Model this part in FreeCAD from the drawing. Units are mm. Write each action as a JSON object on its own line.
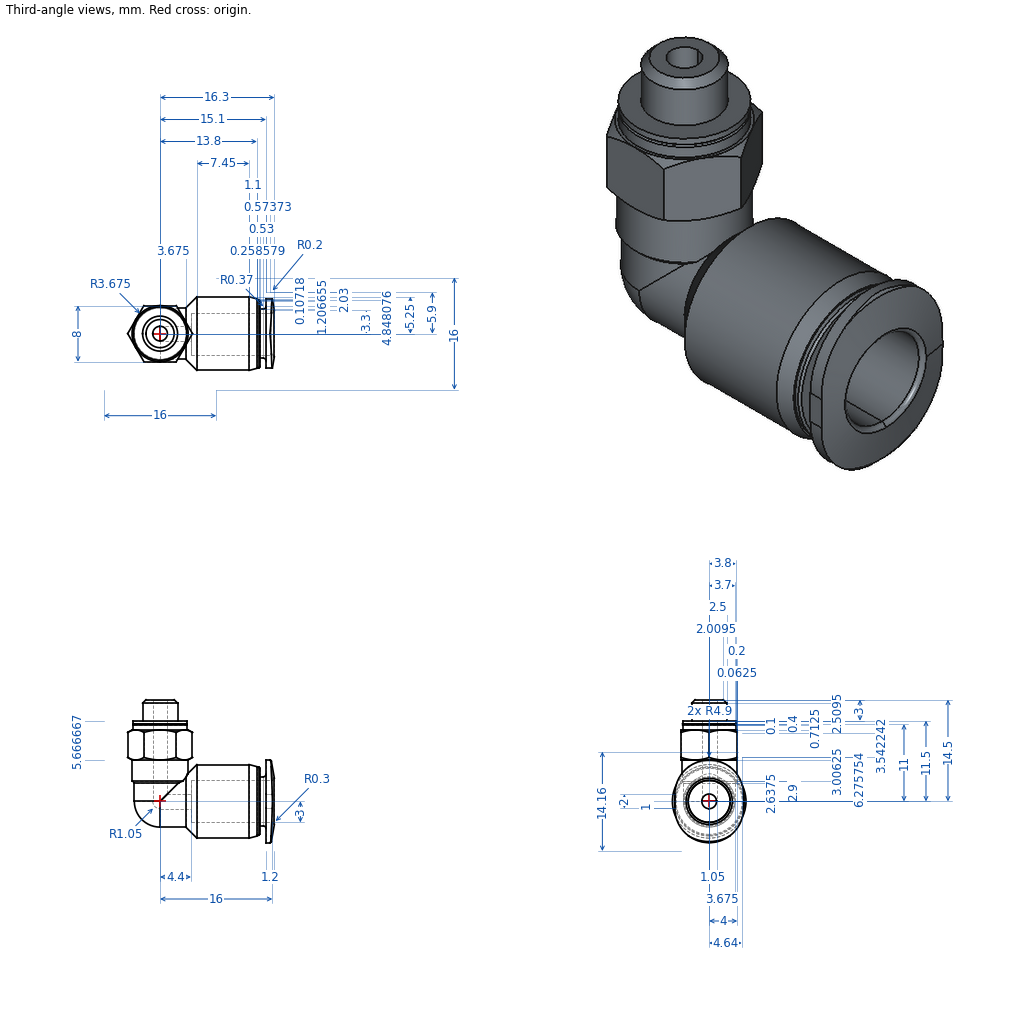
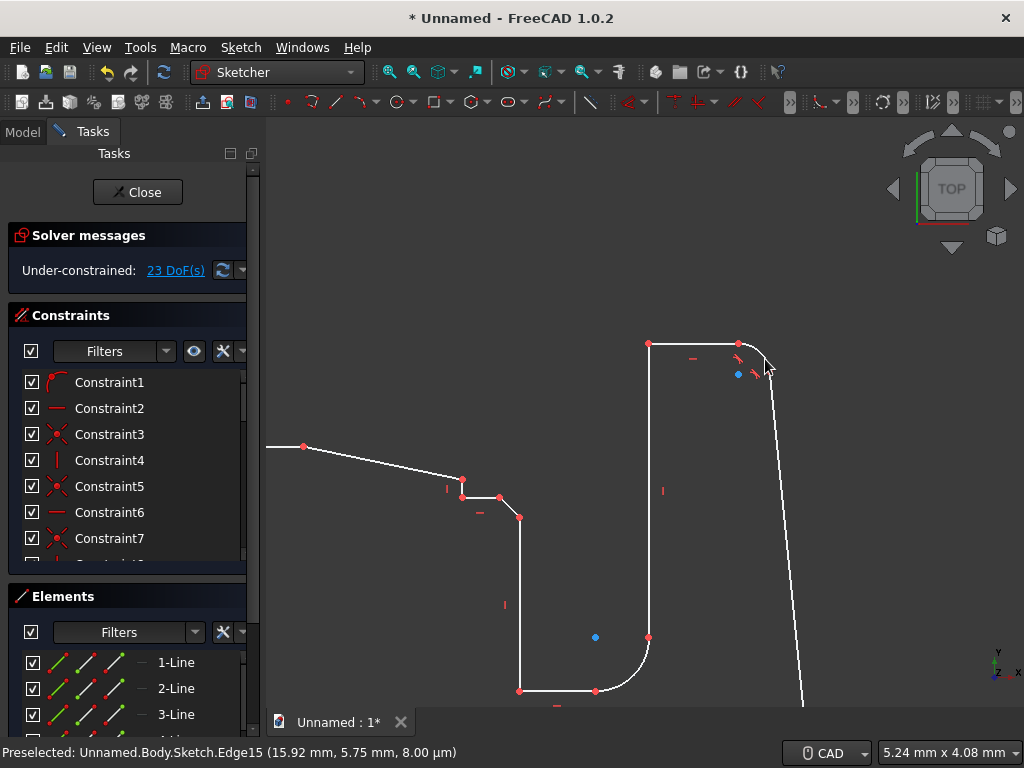
{"action": "scroll", "coordinate": [764, 356], "scroll_direction": "down", "scroll_amount": 10}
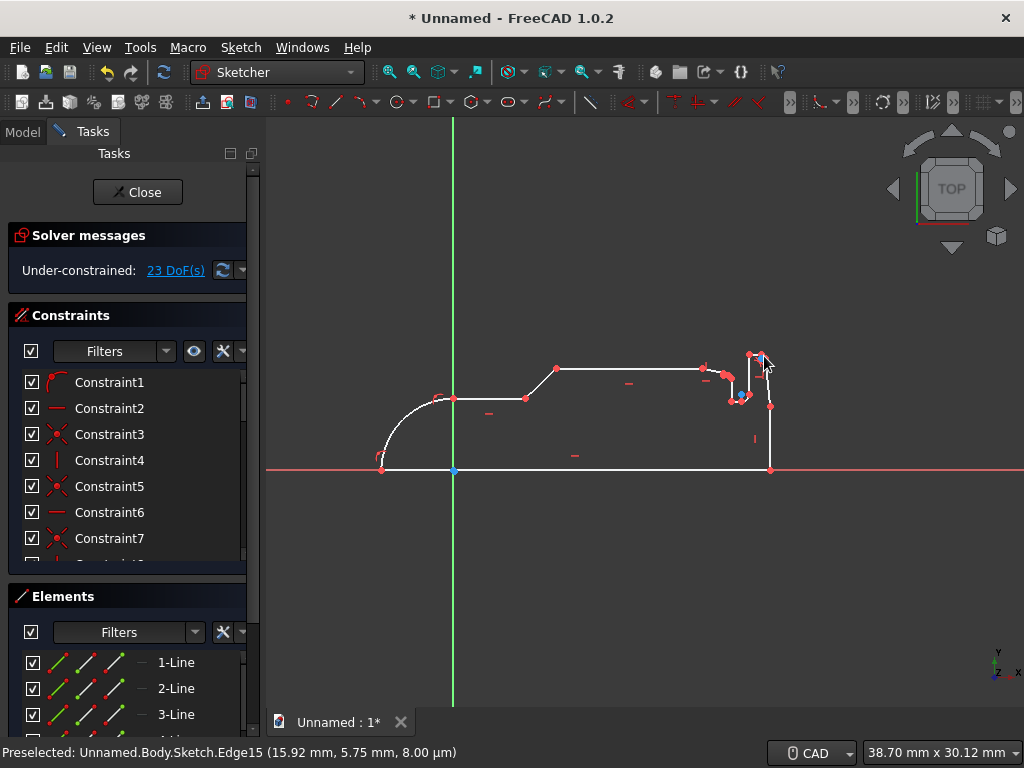
{"action": "left_click", "coordinate": [749, 367]}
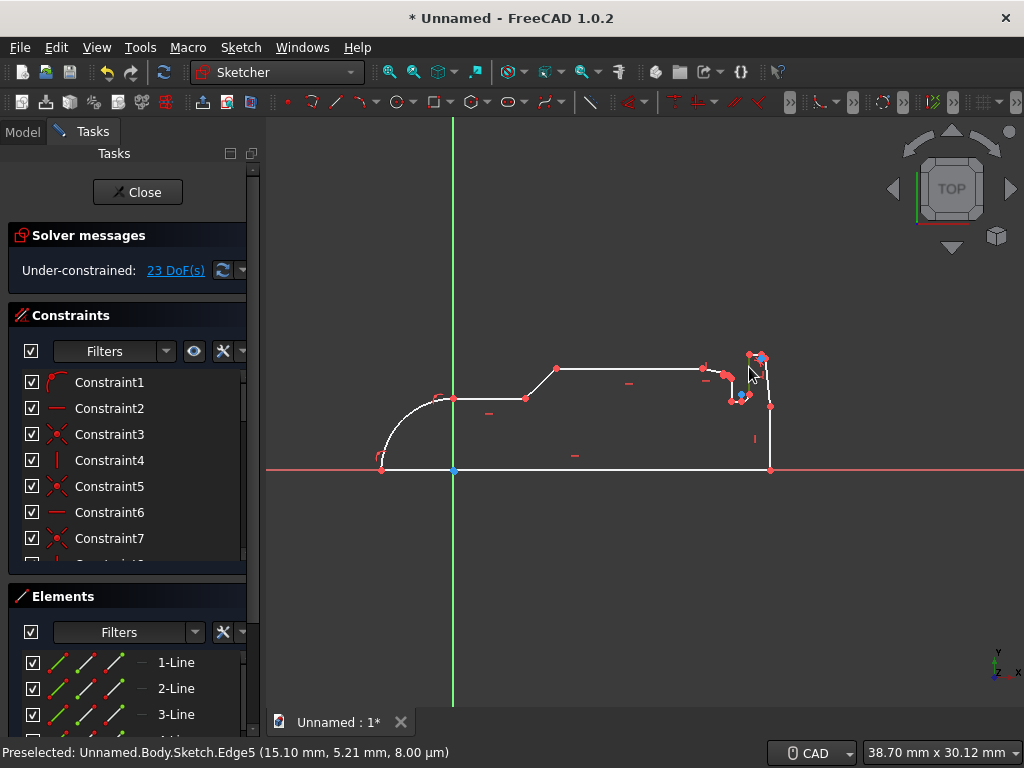
{"action": "scroll", "coordinate": [747, 400], "scroll_direction": "up", "scroll_amount": 5}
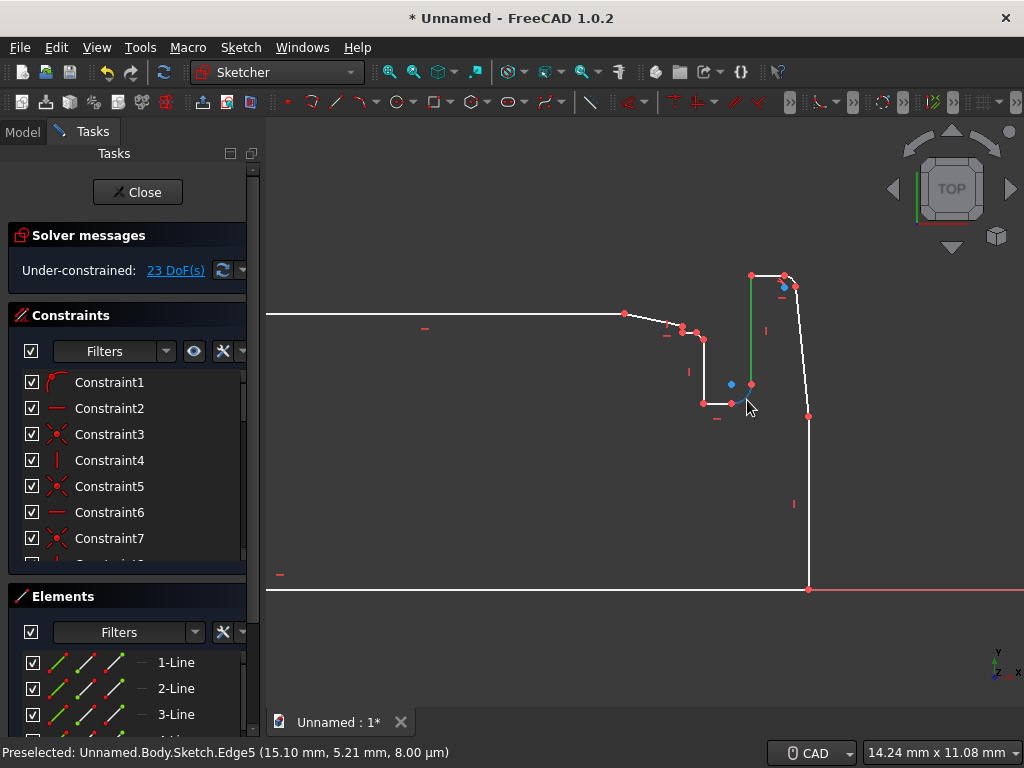
{"action": "left_click", "coordinate": [746, 398]}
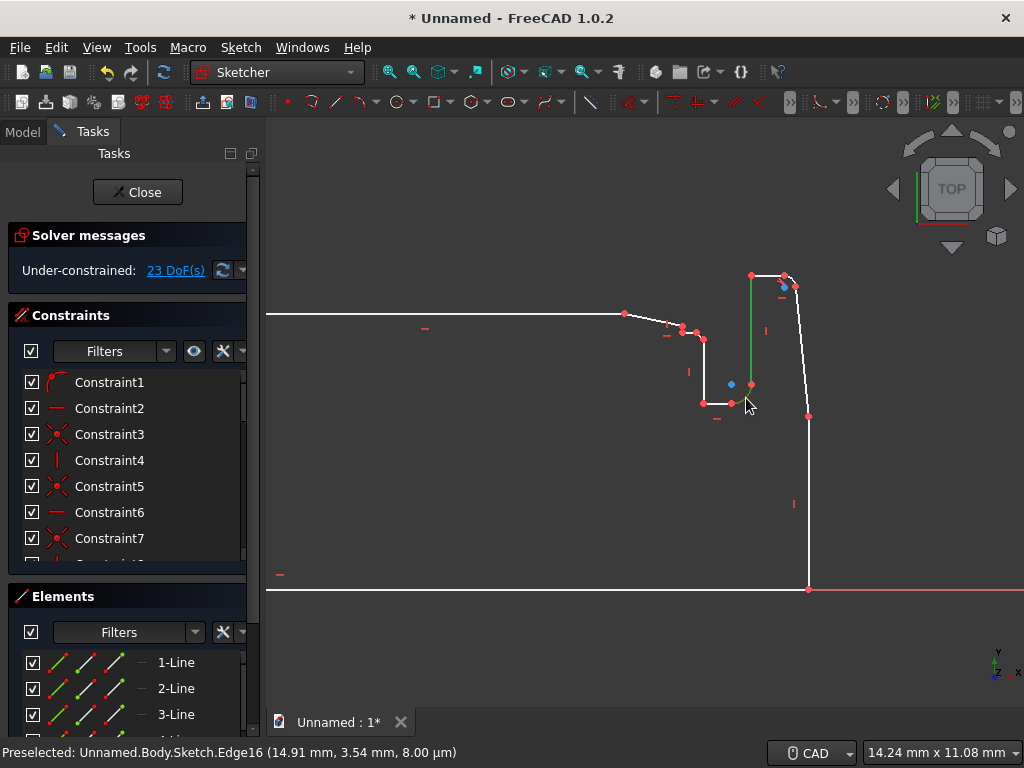
{"action": "key", "text": "t"}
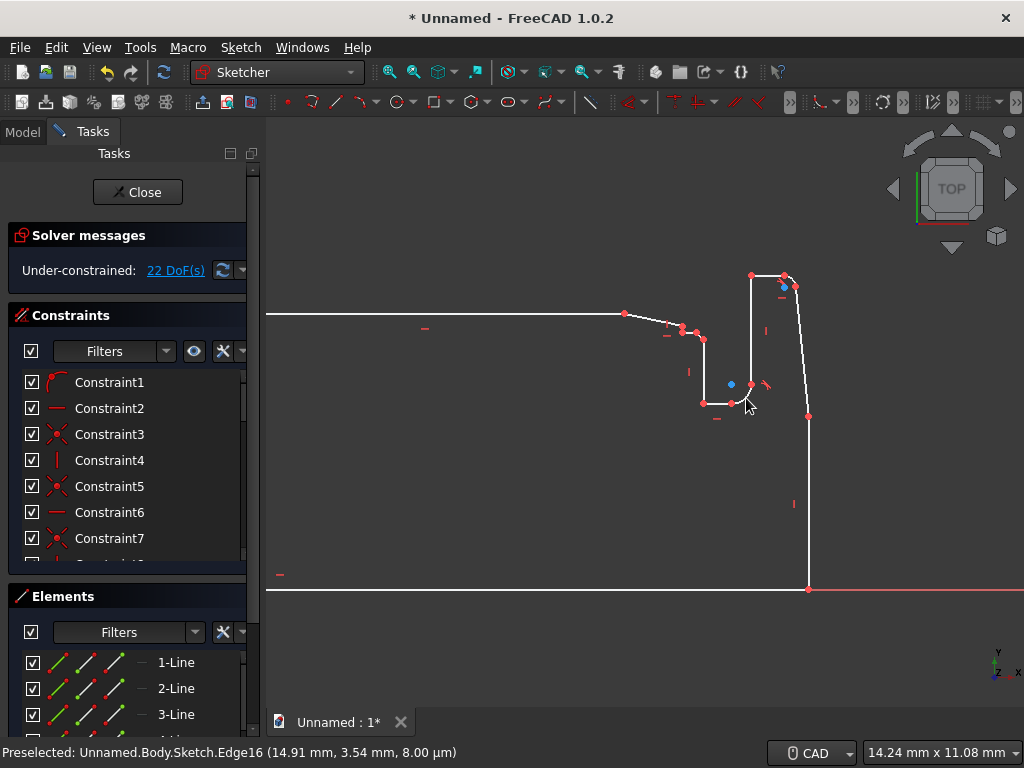
{"action": "scroll", "coordinate": [721, 404], "scroll_direction": "up", "scroll_amount": 2}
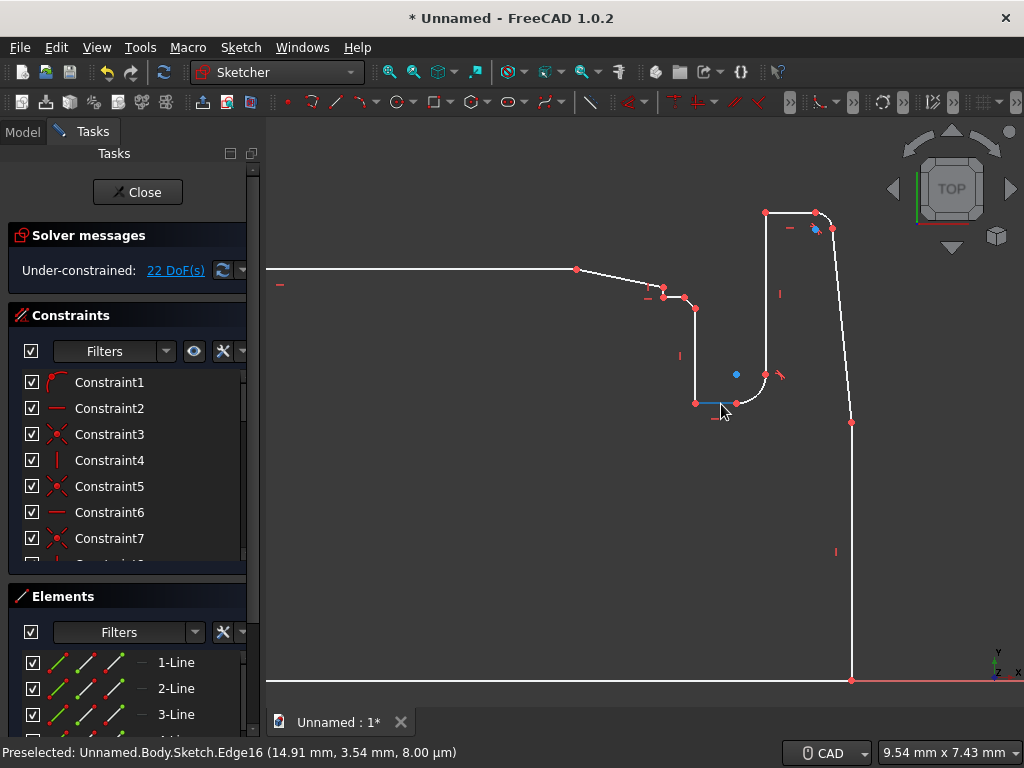
{"action": "left_click", "coordinate": [720, 403]}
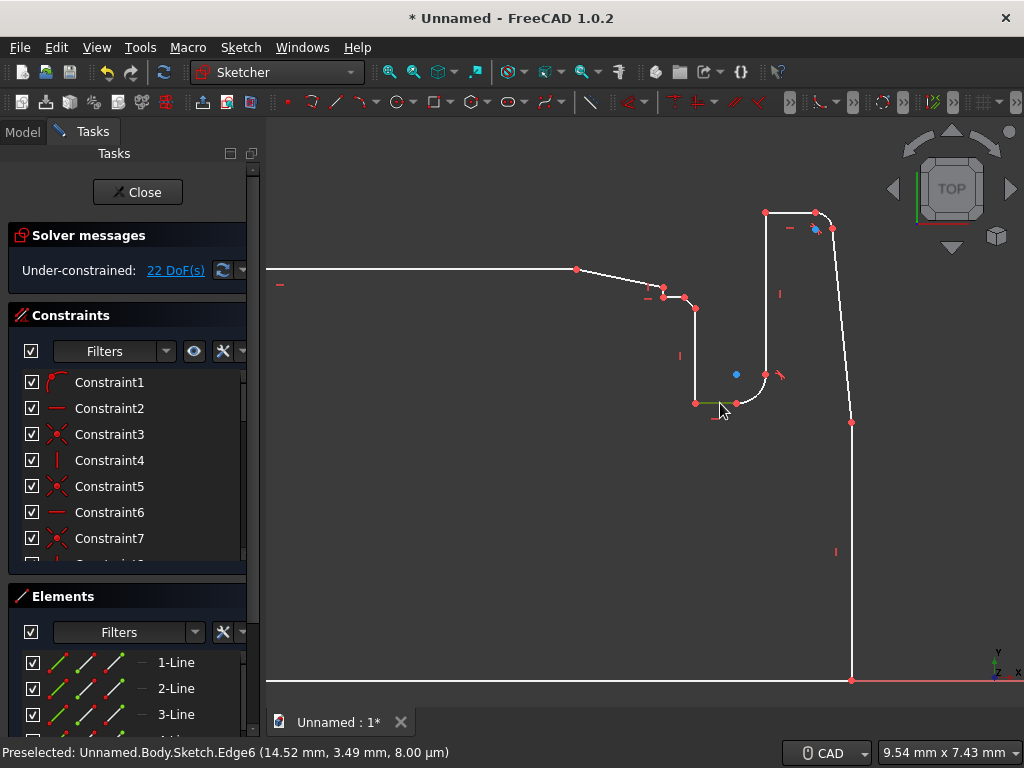
{"action": "left_click", "coordinate": [750, 400]}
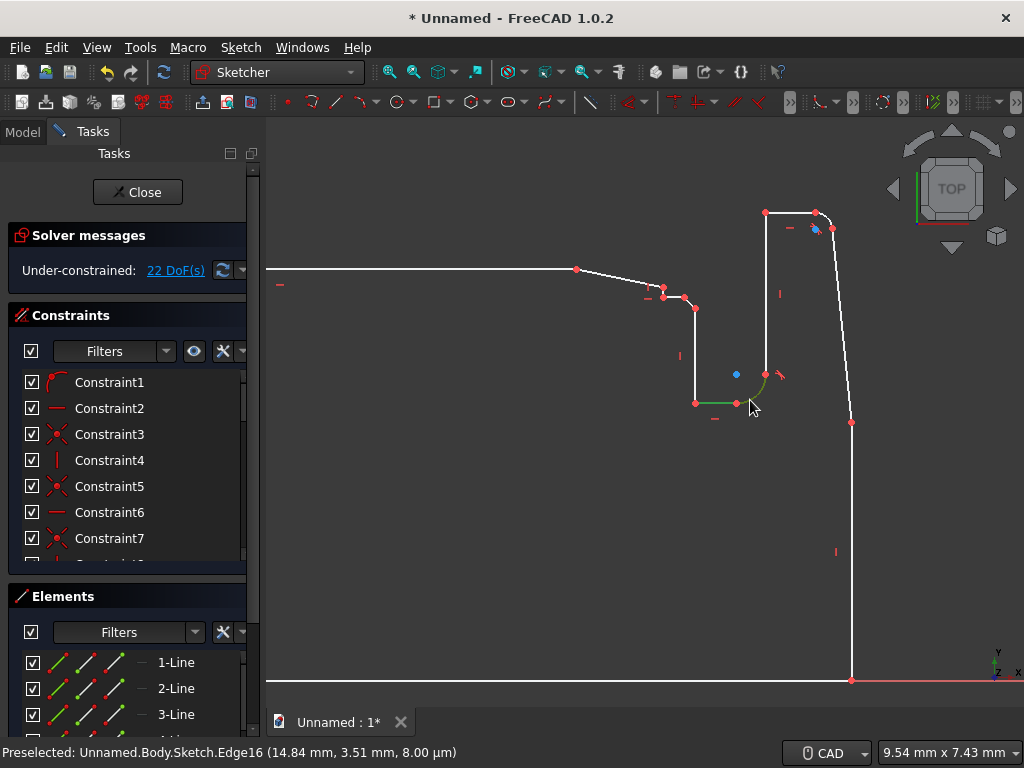
{"action": "key", "text": "t"}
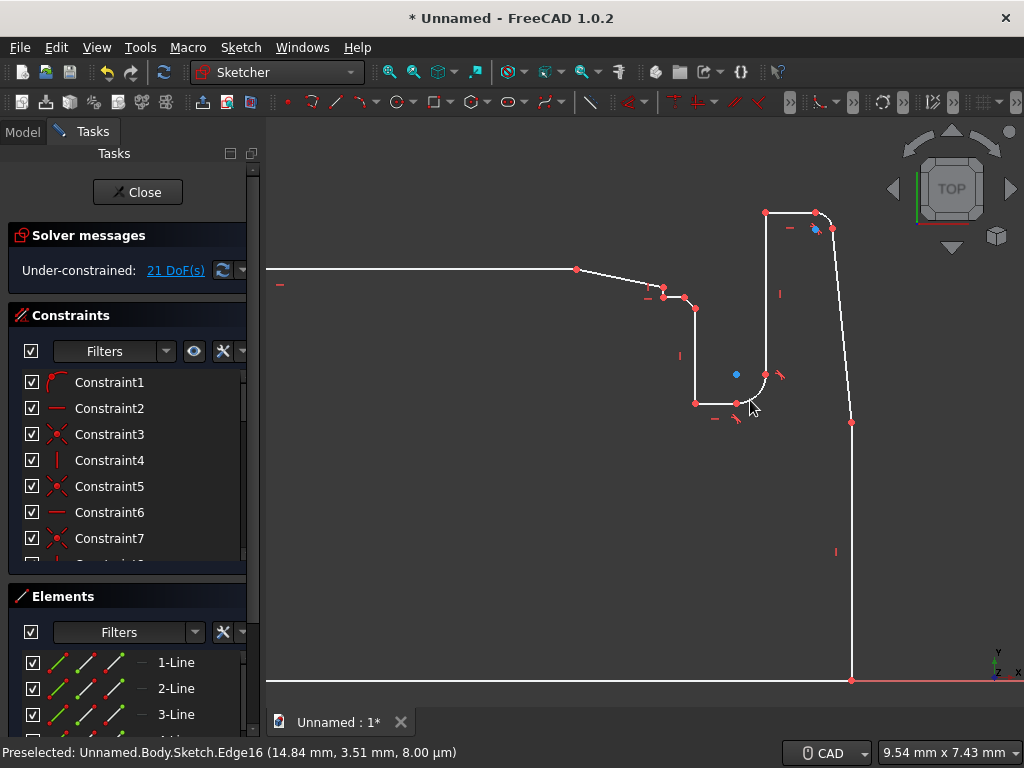
{"action": "scroll", "coordinate": [743, 401], "scroll_direction": "down", "scroll_amount": 7}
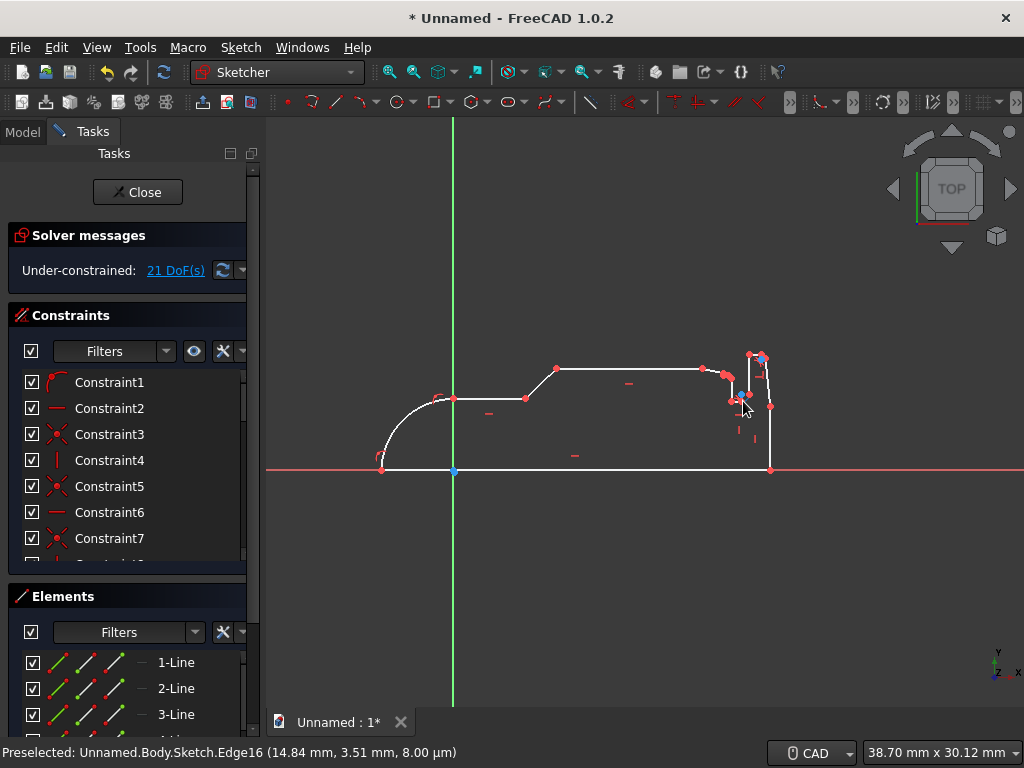
{"action": "left_click", "coordinate": [504, 399]}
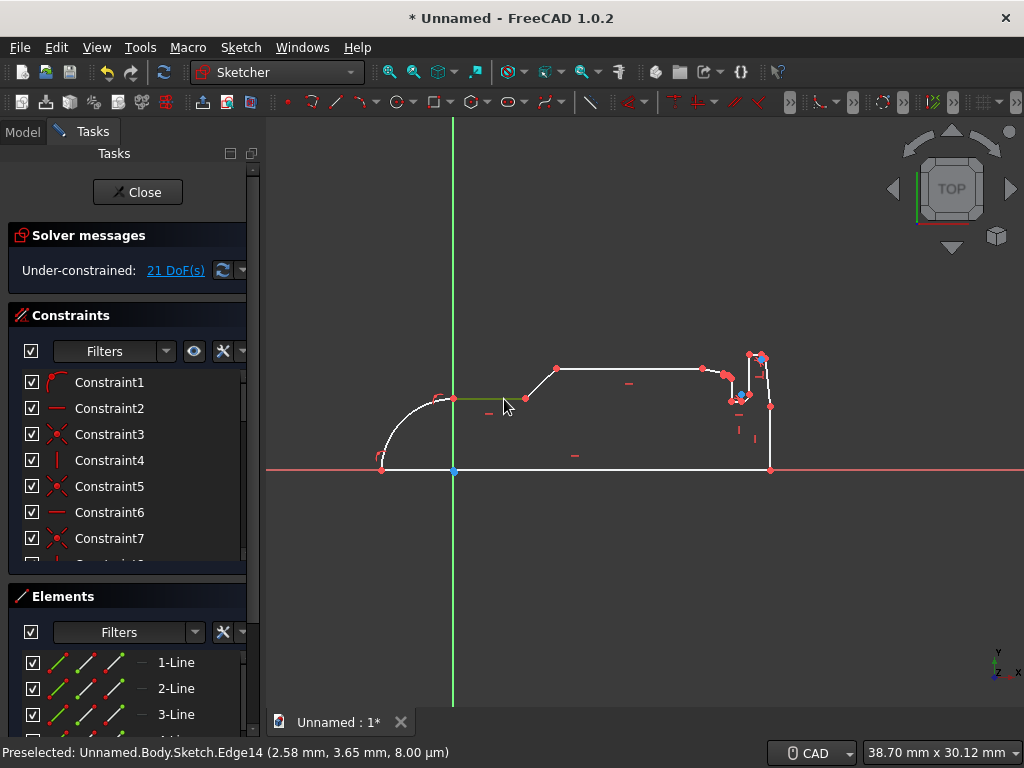
{"action": "left_click", "coordinate": [421, 407]}